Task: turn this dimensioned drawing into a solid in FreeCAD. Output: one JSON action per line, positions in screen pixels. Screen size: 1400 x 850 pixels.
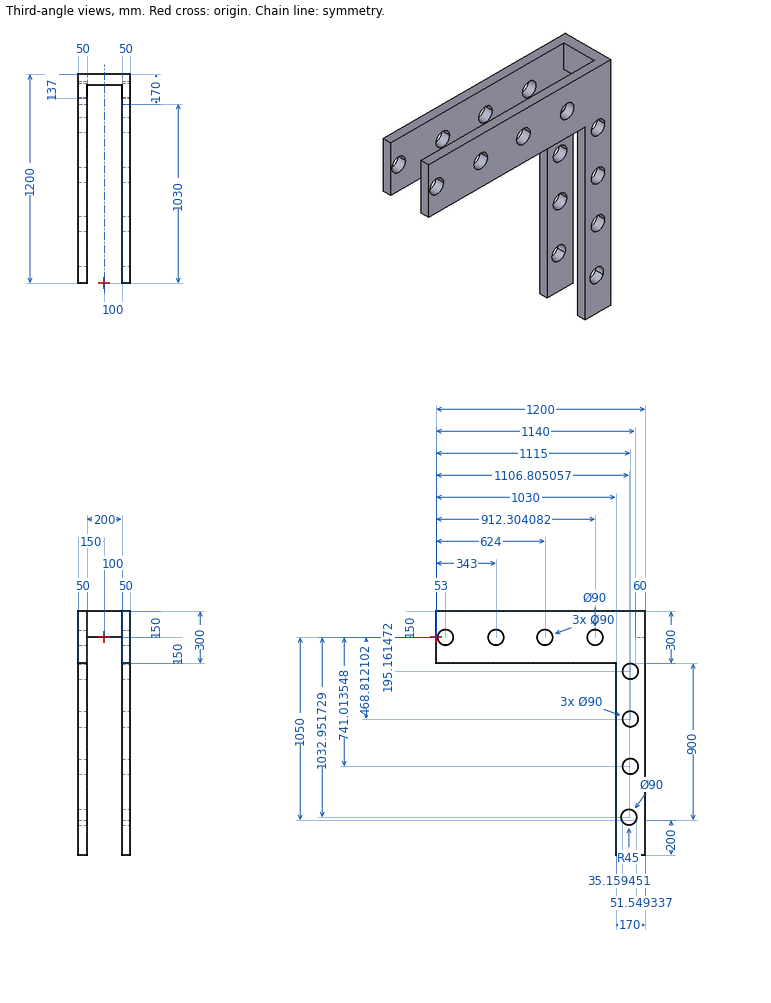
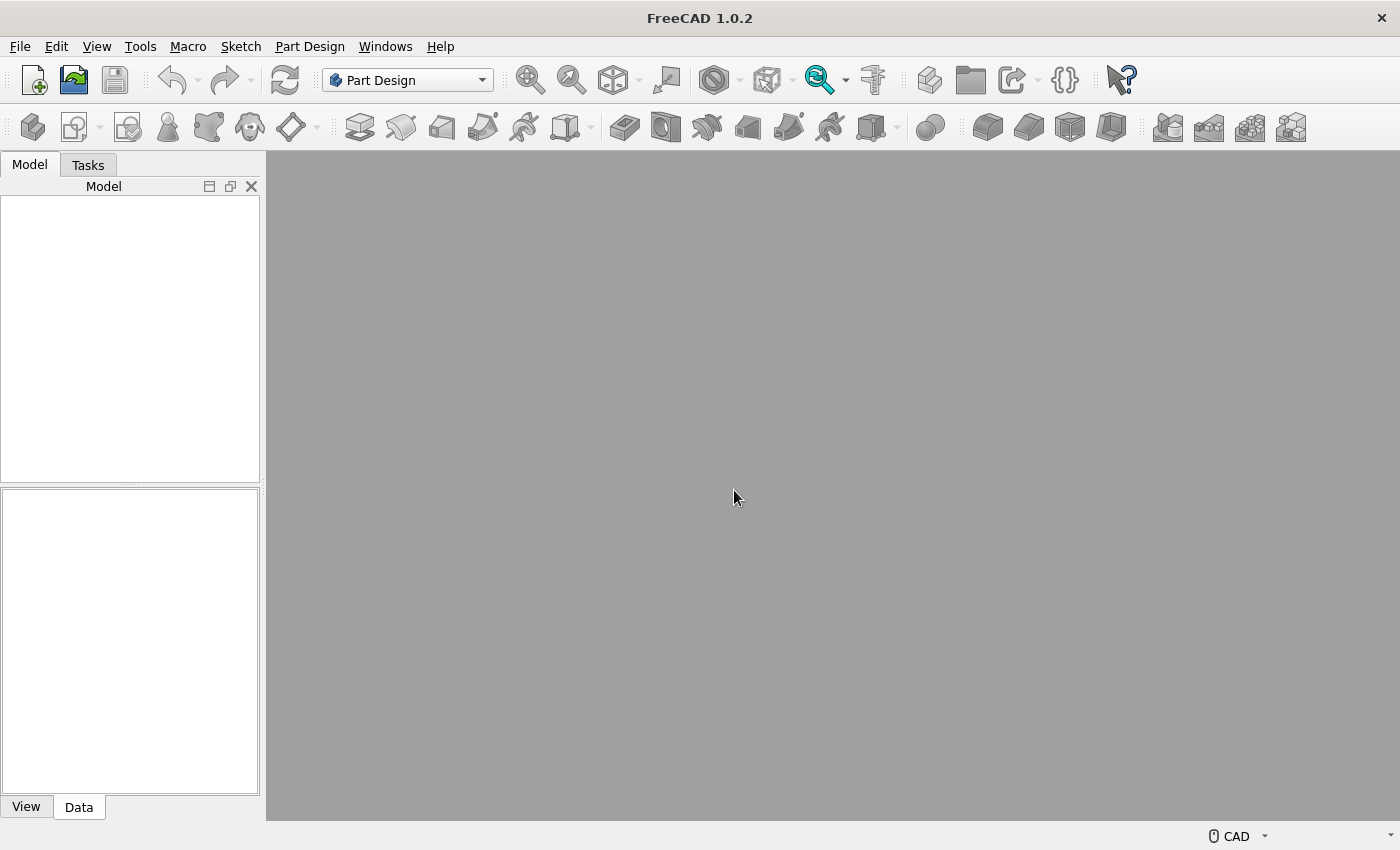
{"action": "left_click", "coordinate": [33, 80]}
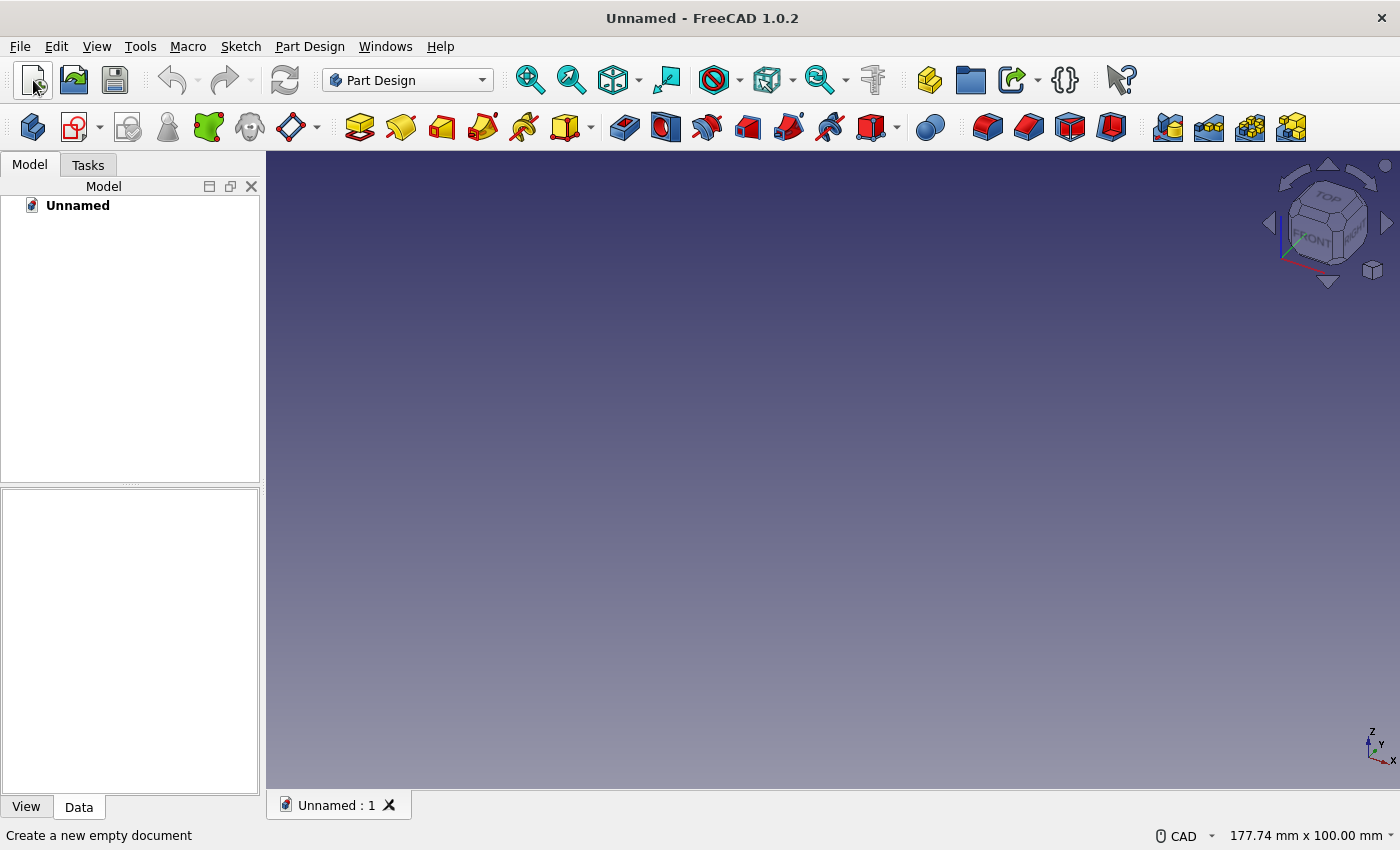
{"action": "left_click", "coordinate": [74, 128]}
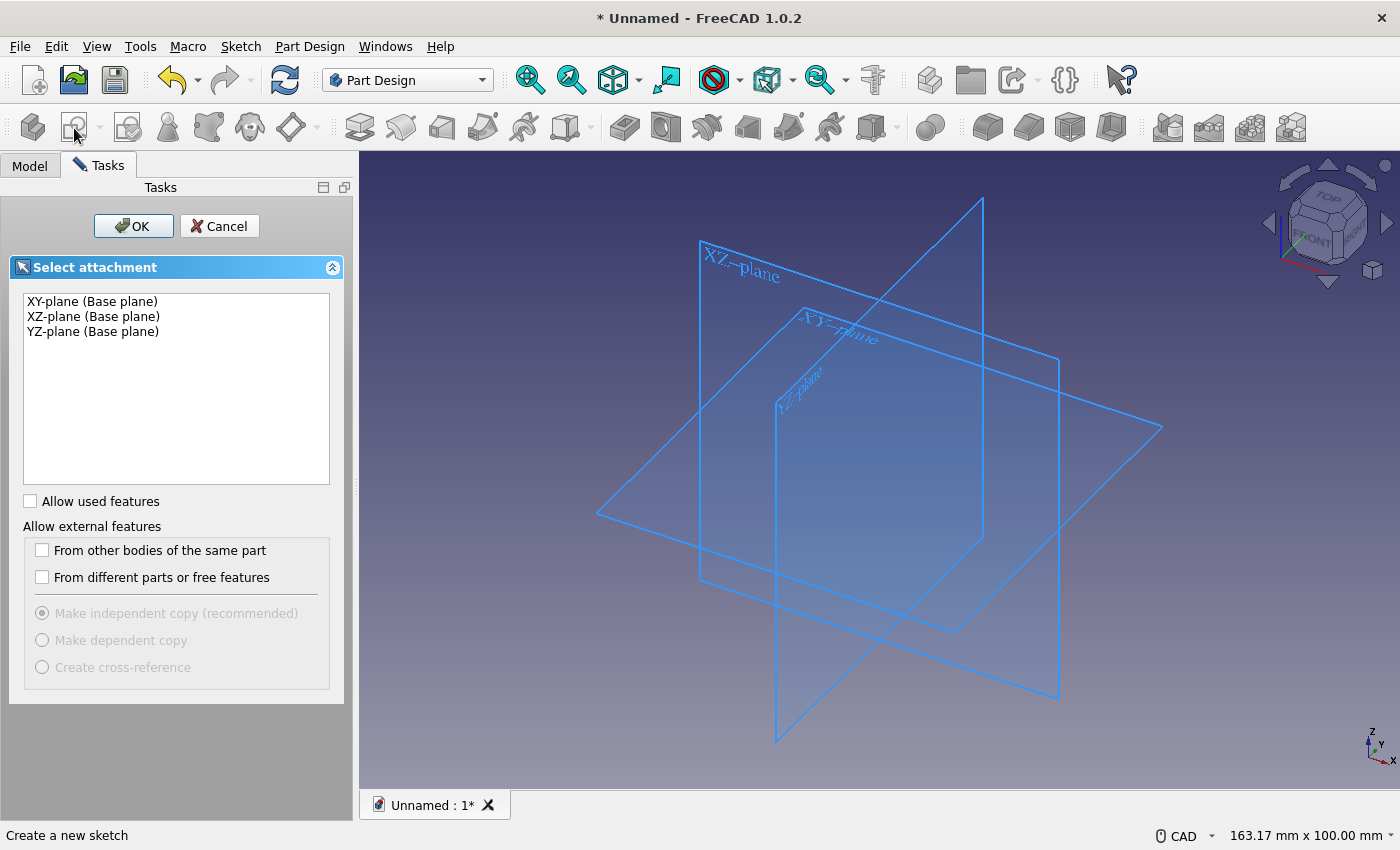
{"action": "left_click", "coordinate": [84, 316]}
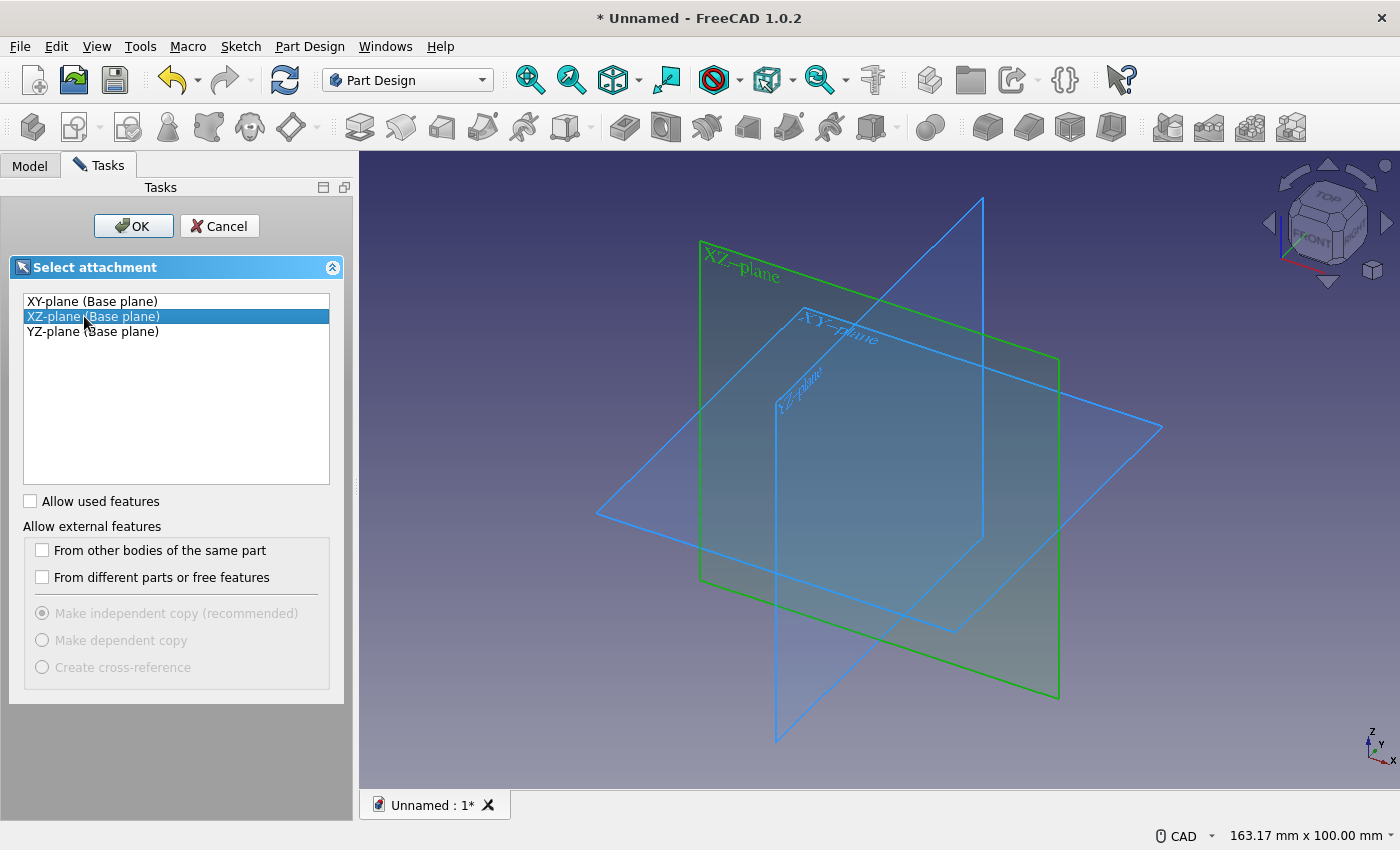
{"action": "left_click", "coordinate": [134, 226]}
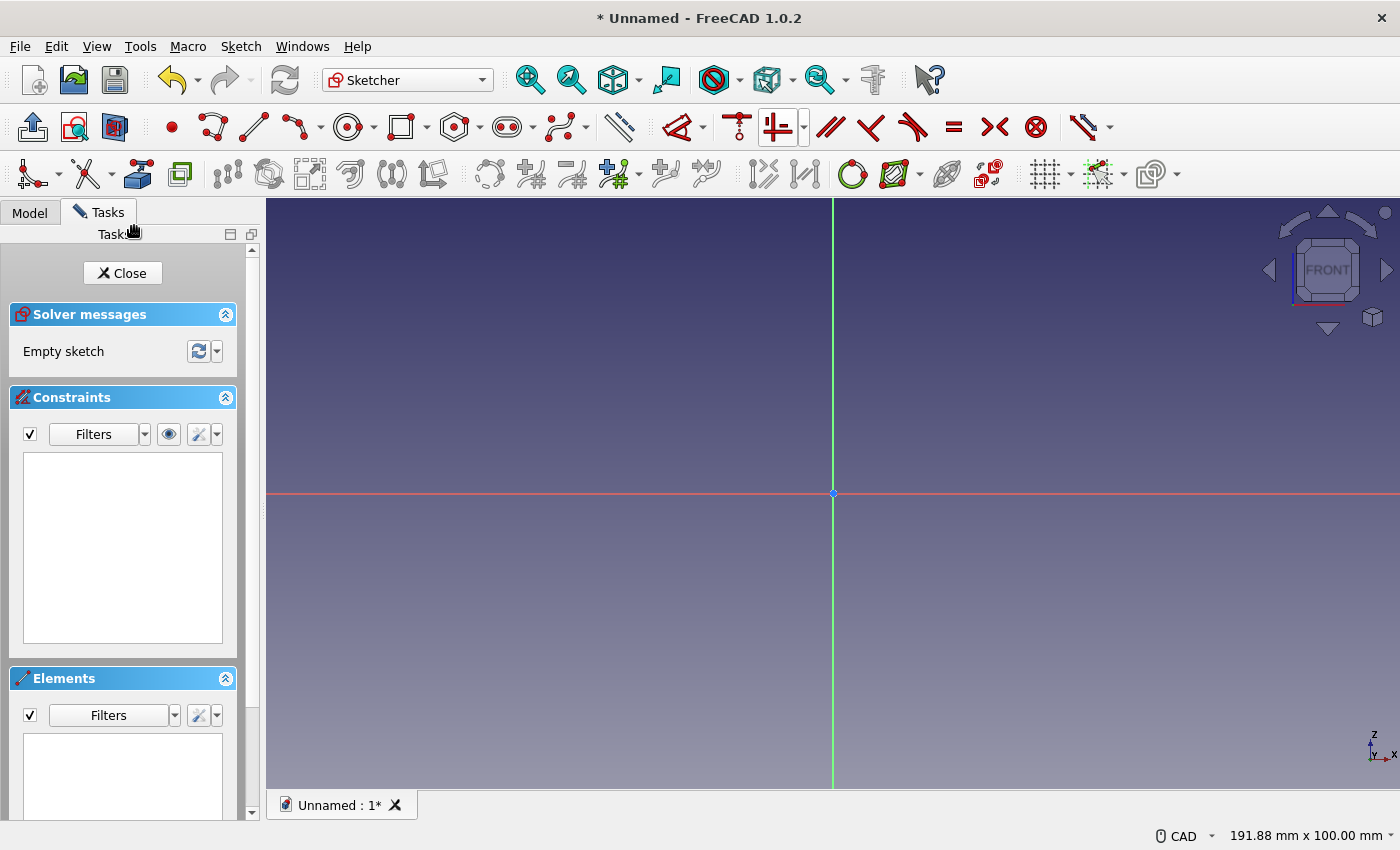
{"action": "scroll", "coordinate": [635, 493], "scroll_direction": "down", "scroll_amount": 8}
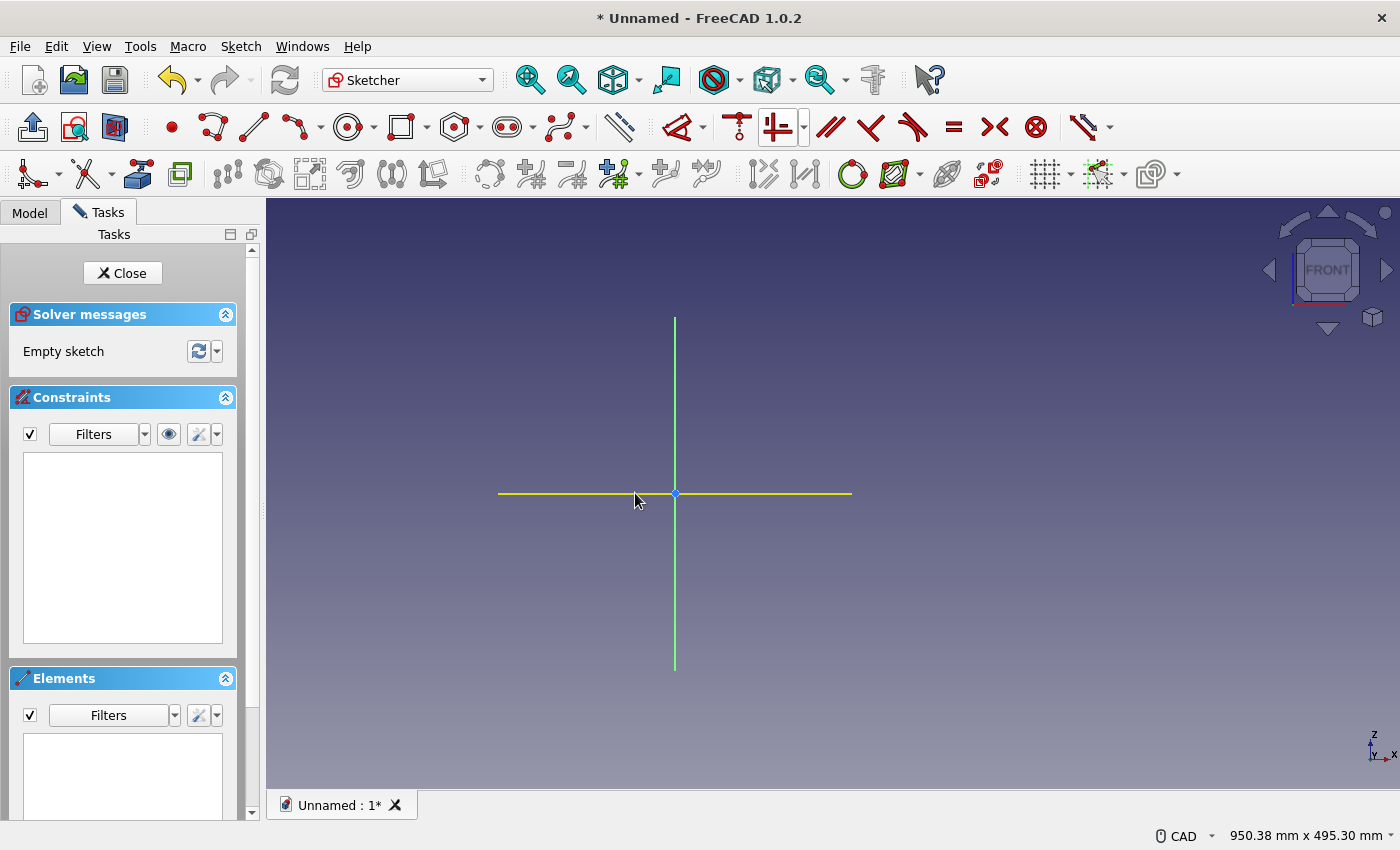
{"action": "left_click", "coordinate": [400, 128]}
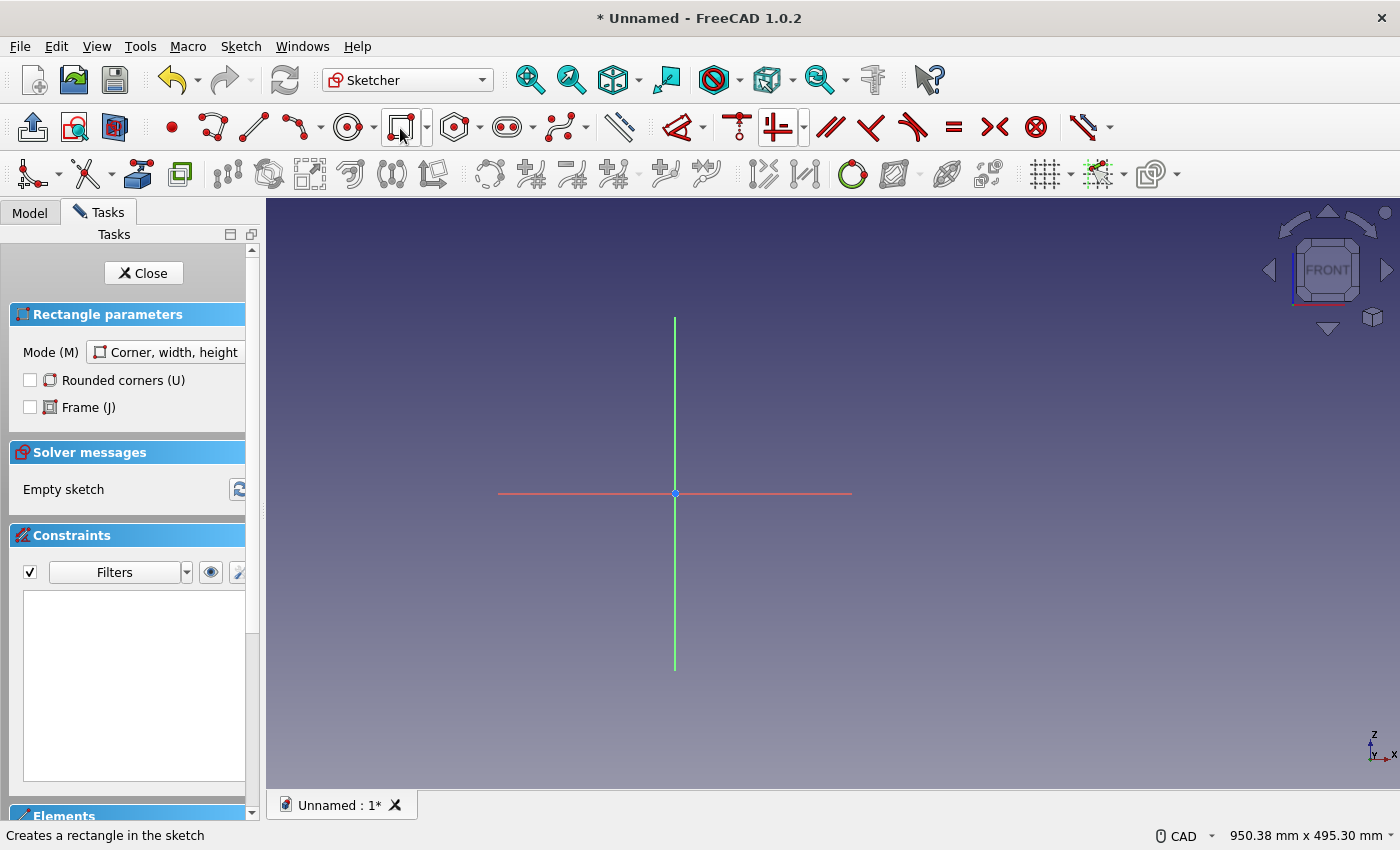
{"action": "left_click", "coordinate": [795, 315]}
{"action": "left_click", "coordinate": [854, 672]}
{"action": "key", "text": "Escape"}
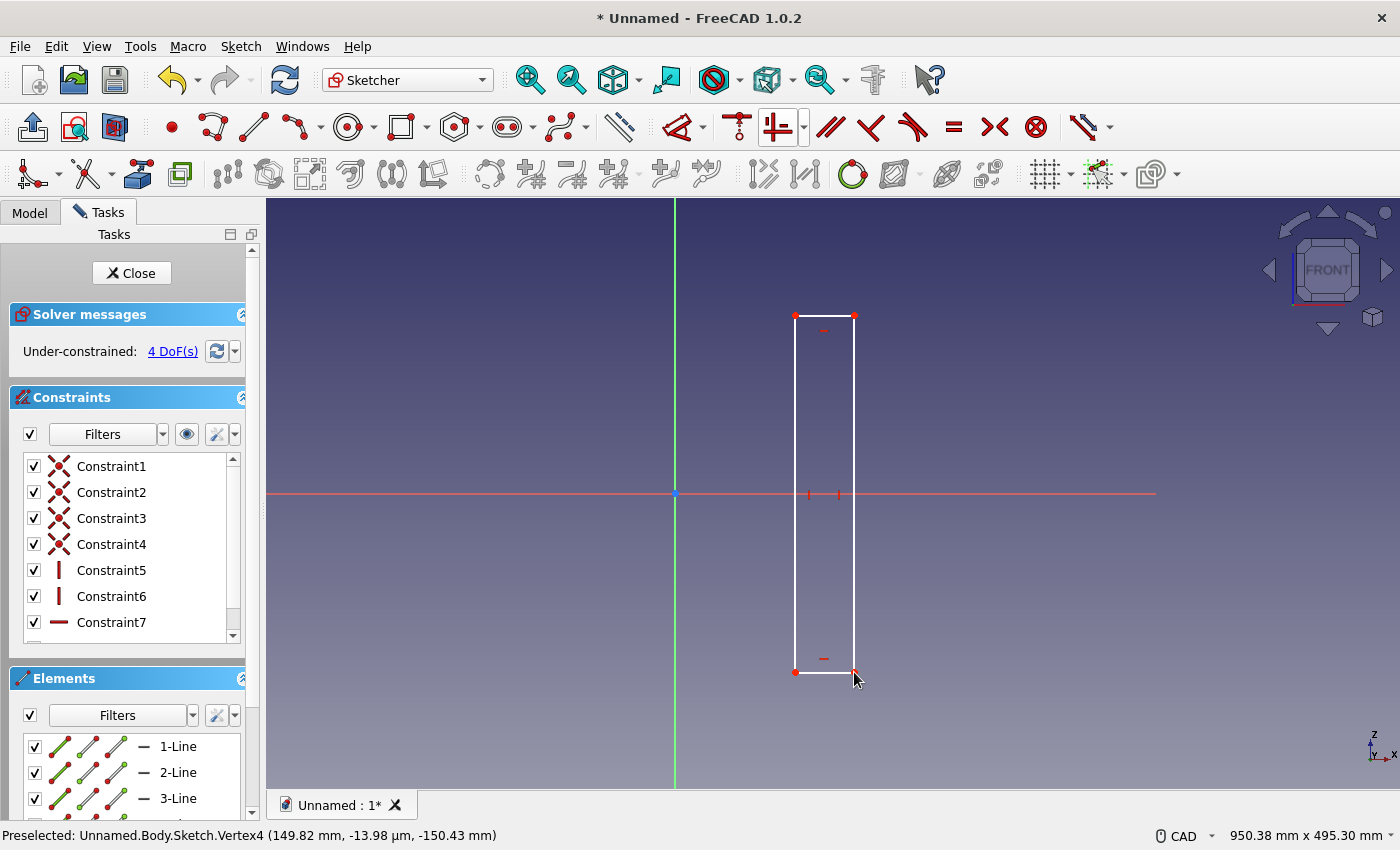
{"action": "left_click", "coordinate": [813, 673]}